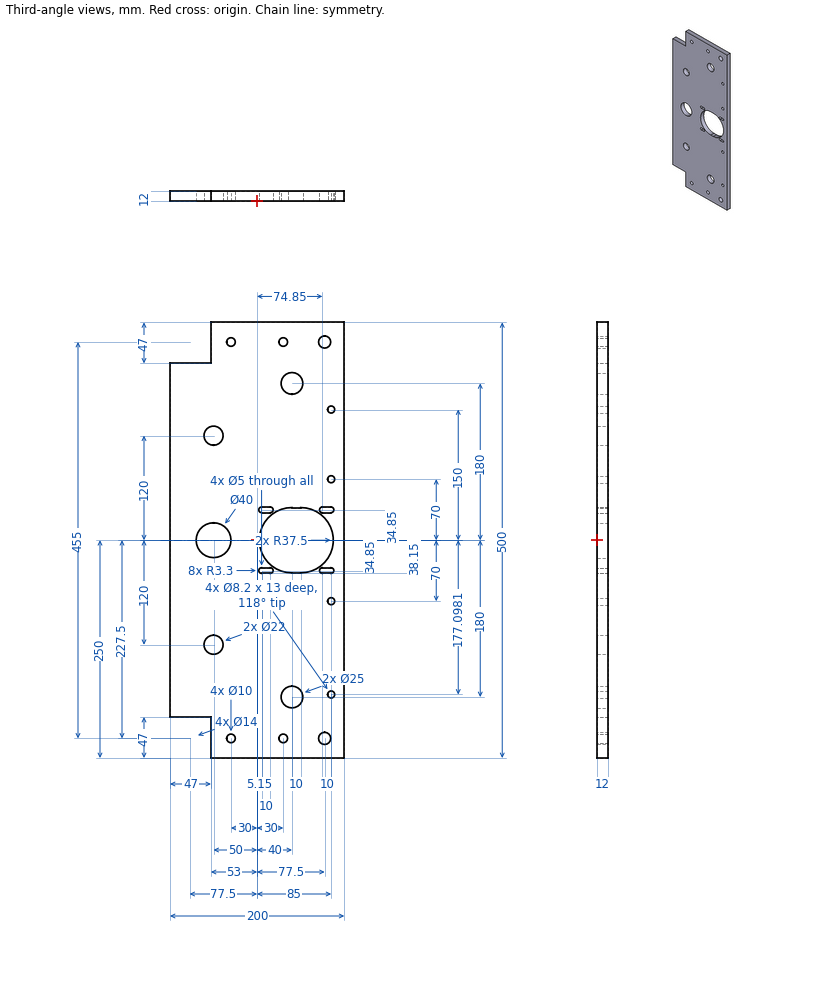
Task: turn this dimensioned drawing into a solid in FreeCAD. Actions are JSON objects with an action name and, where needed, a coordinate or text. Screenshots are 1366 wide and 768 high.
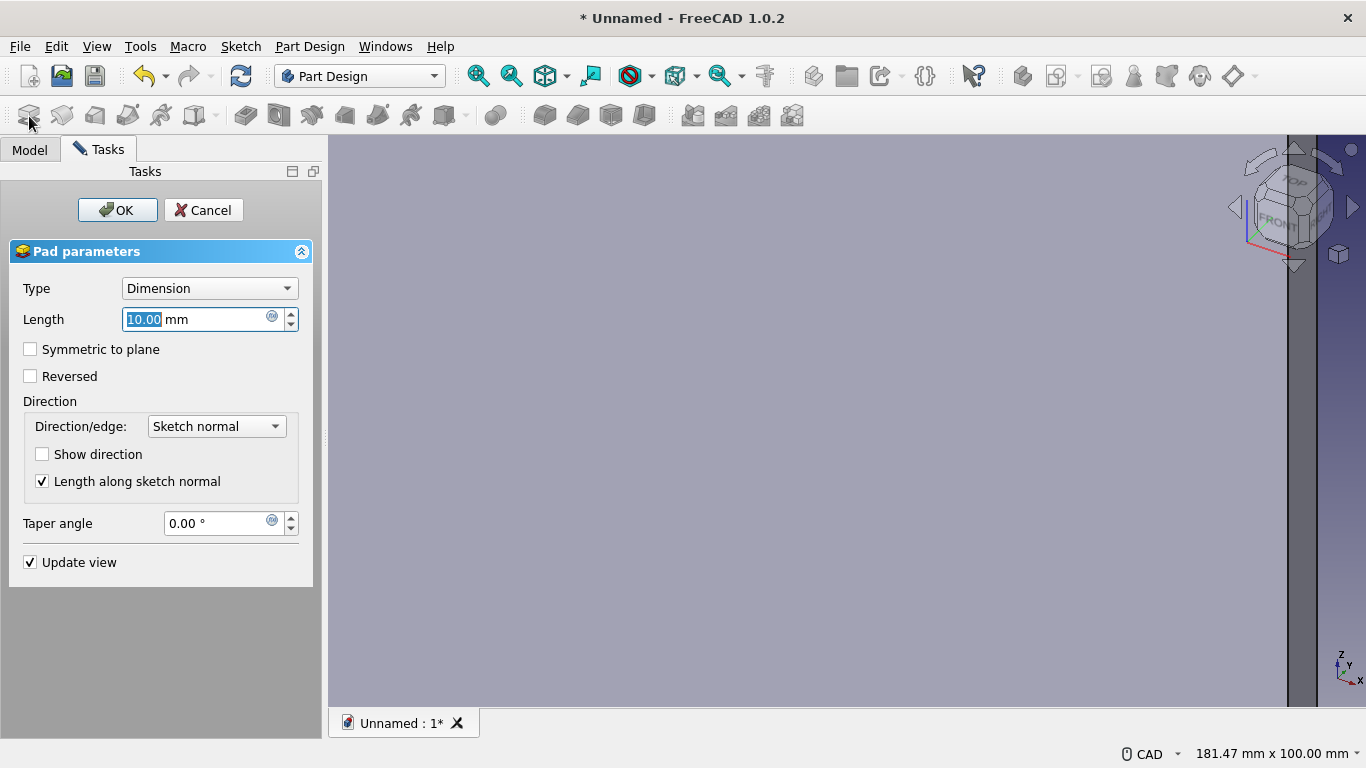
{"action": "type", "text": "12"}
{"action": "key", "text": "Tab"}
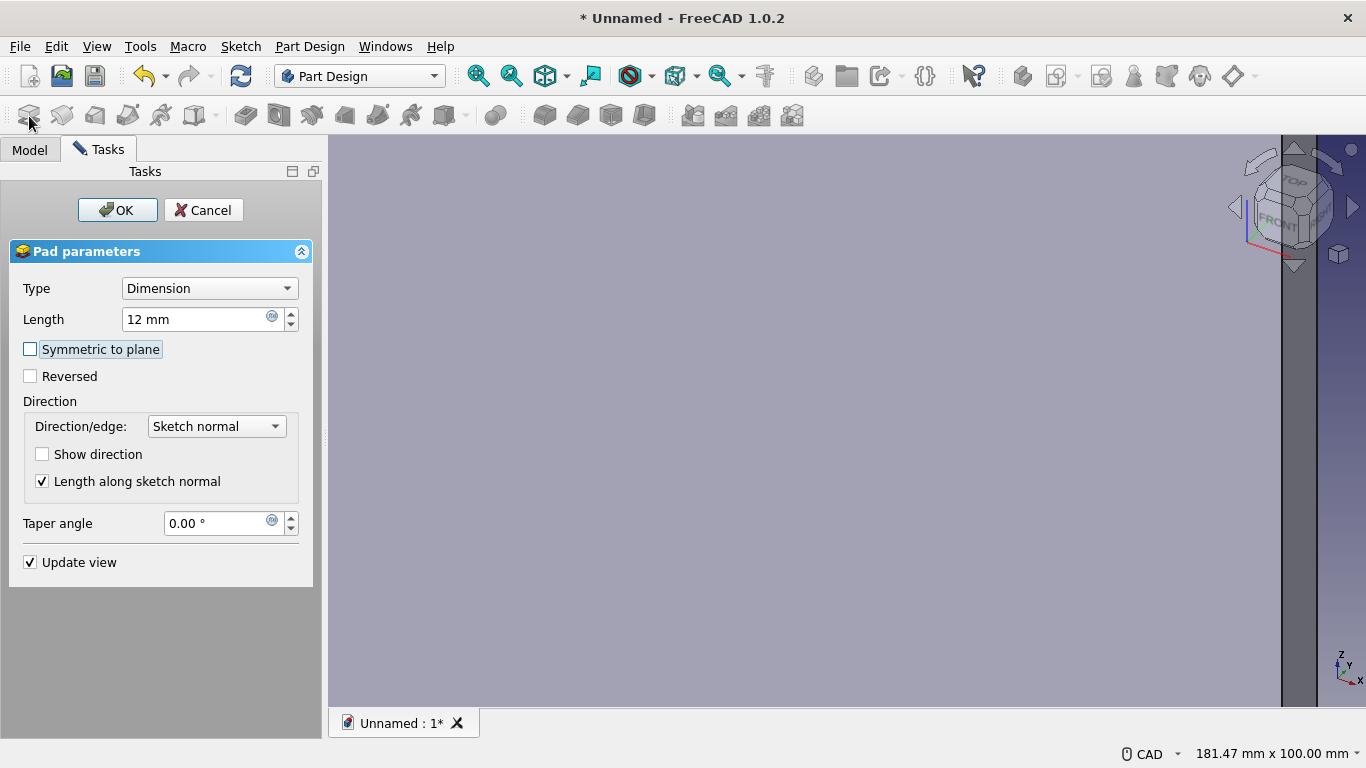
{"action": "left_click", "coordinate": [31, 376]}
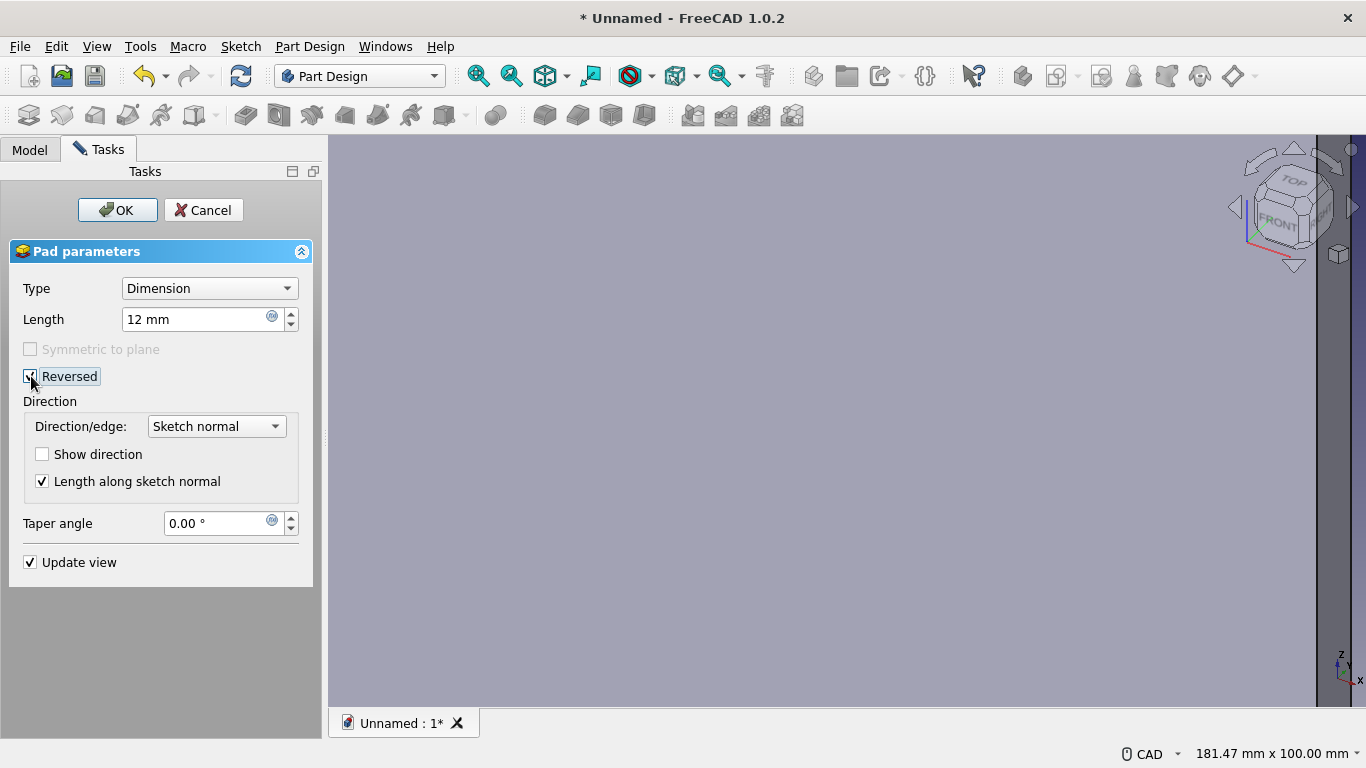
{"action": "left_click", "coordinate": [118, 210]}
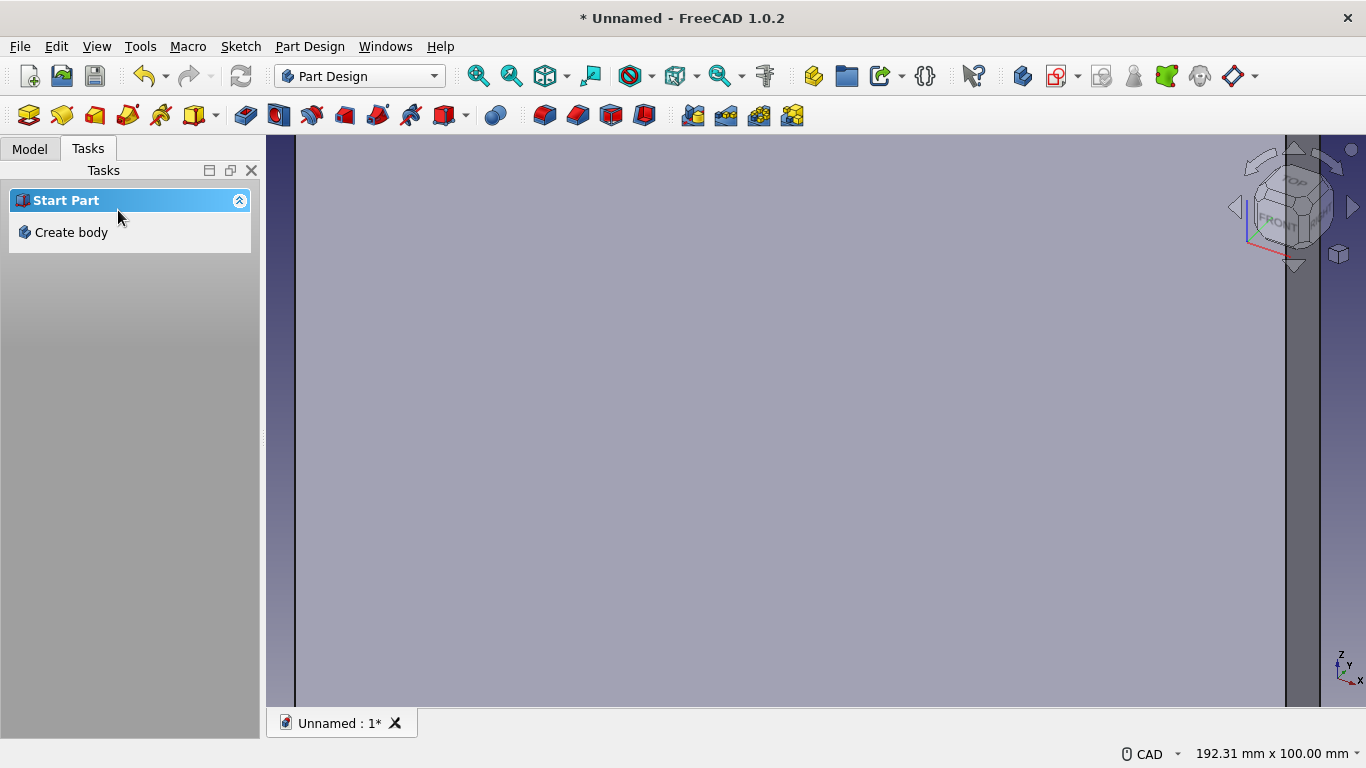
{"action": "key", "text": "v f"}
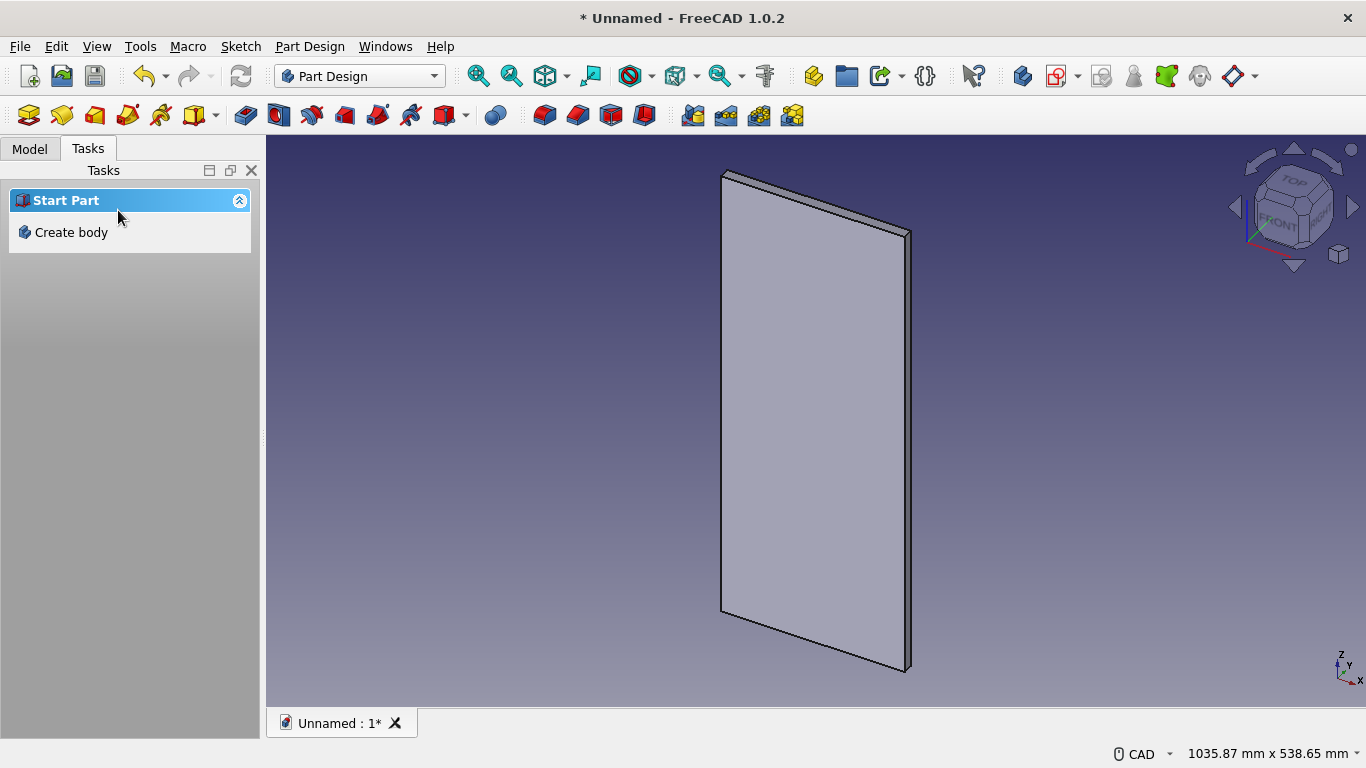
{"action": "key", "text": "4"}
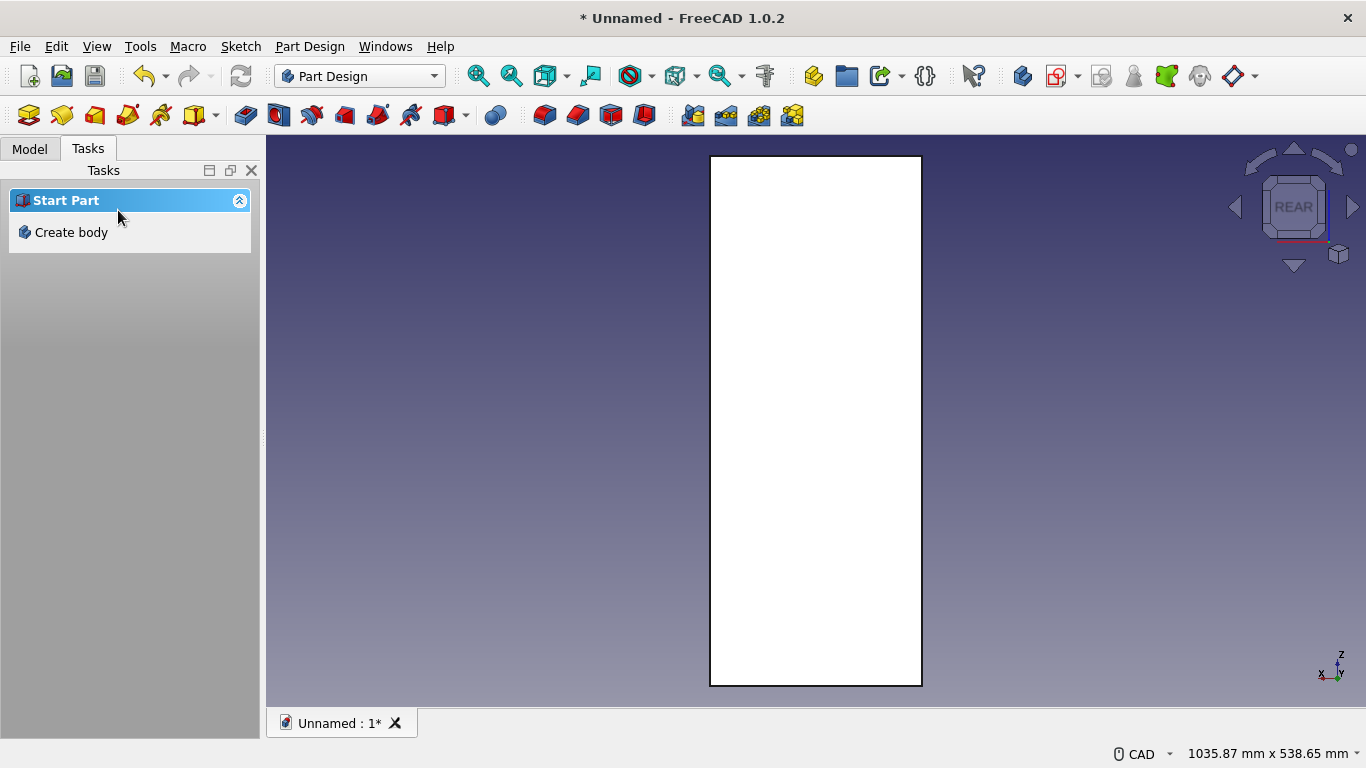
{"action": "left_click", "coordinate": [816, 268]}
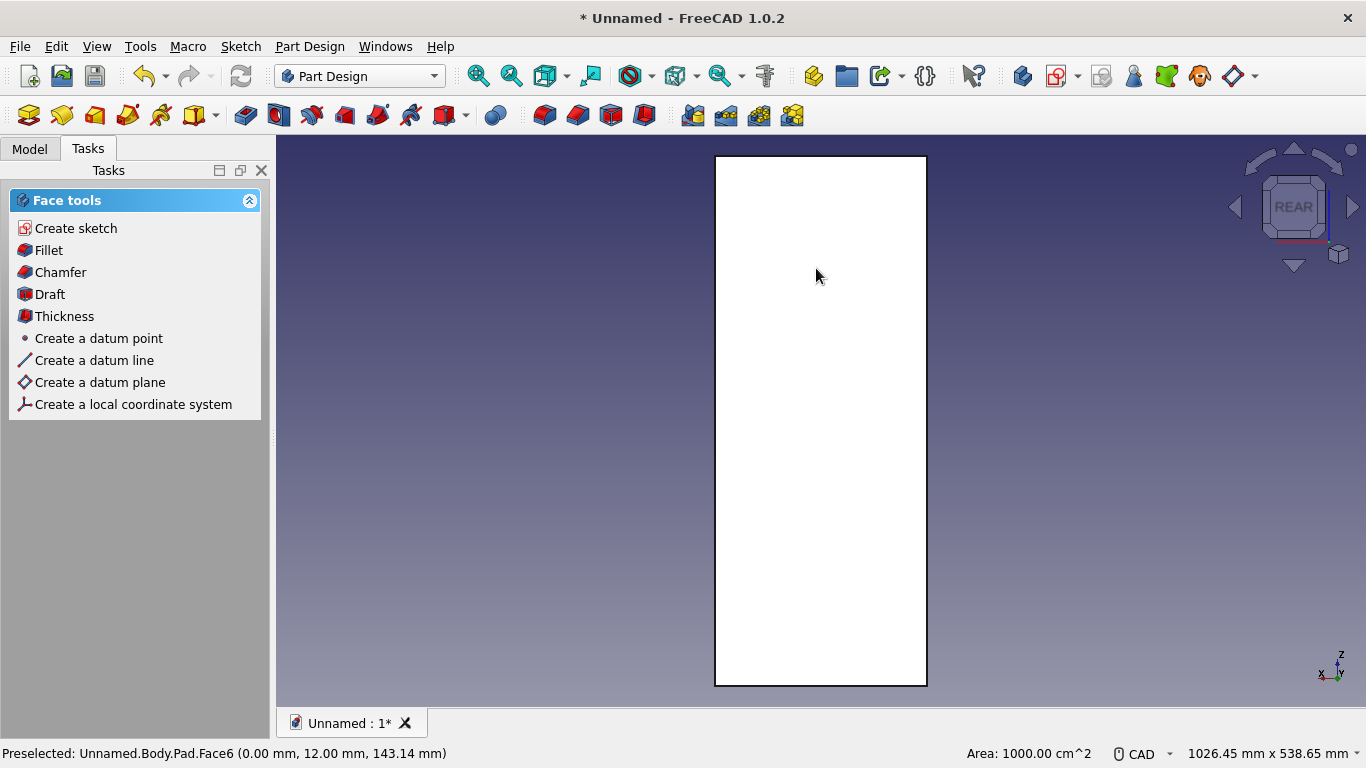
{"action": "left_click", "coordinate": [1056, 76]}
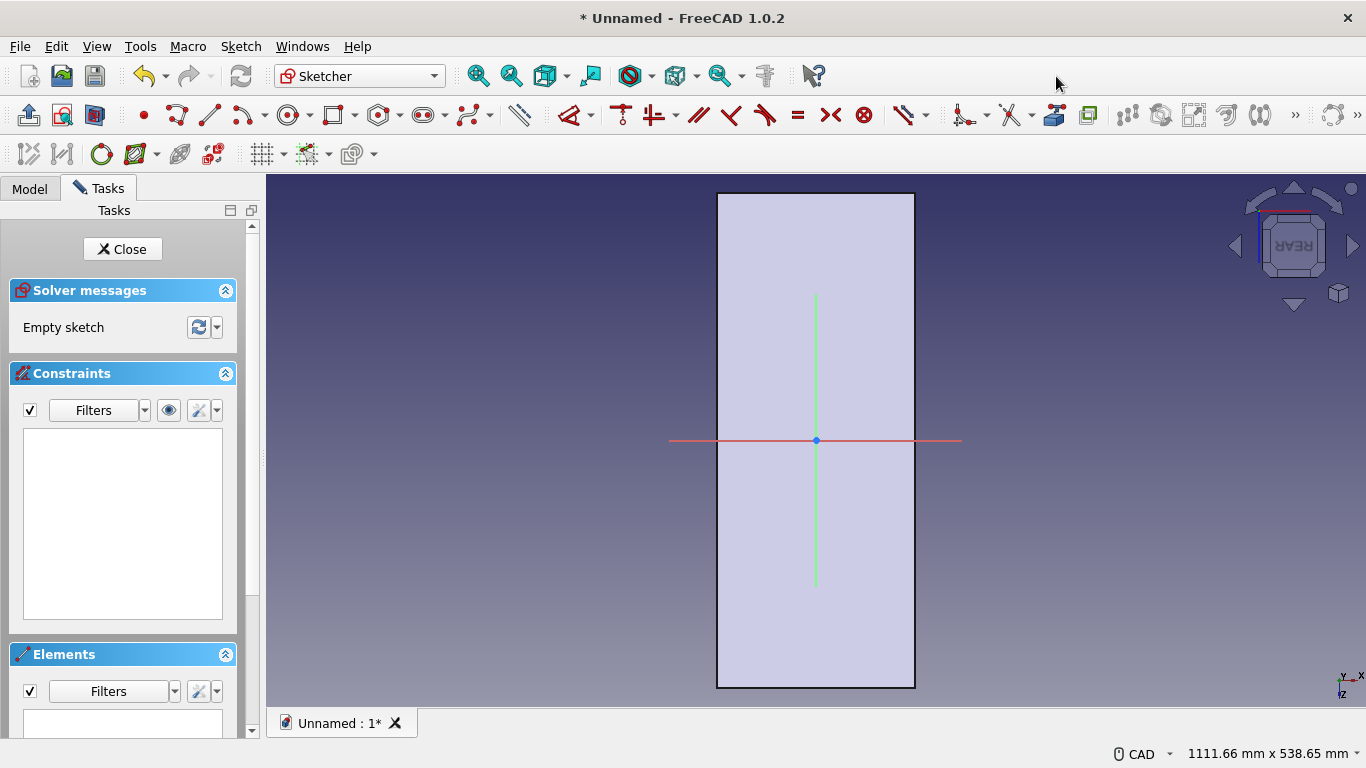
{"action": "key", "text": "g c"}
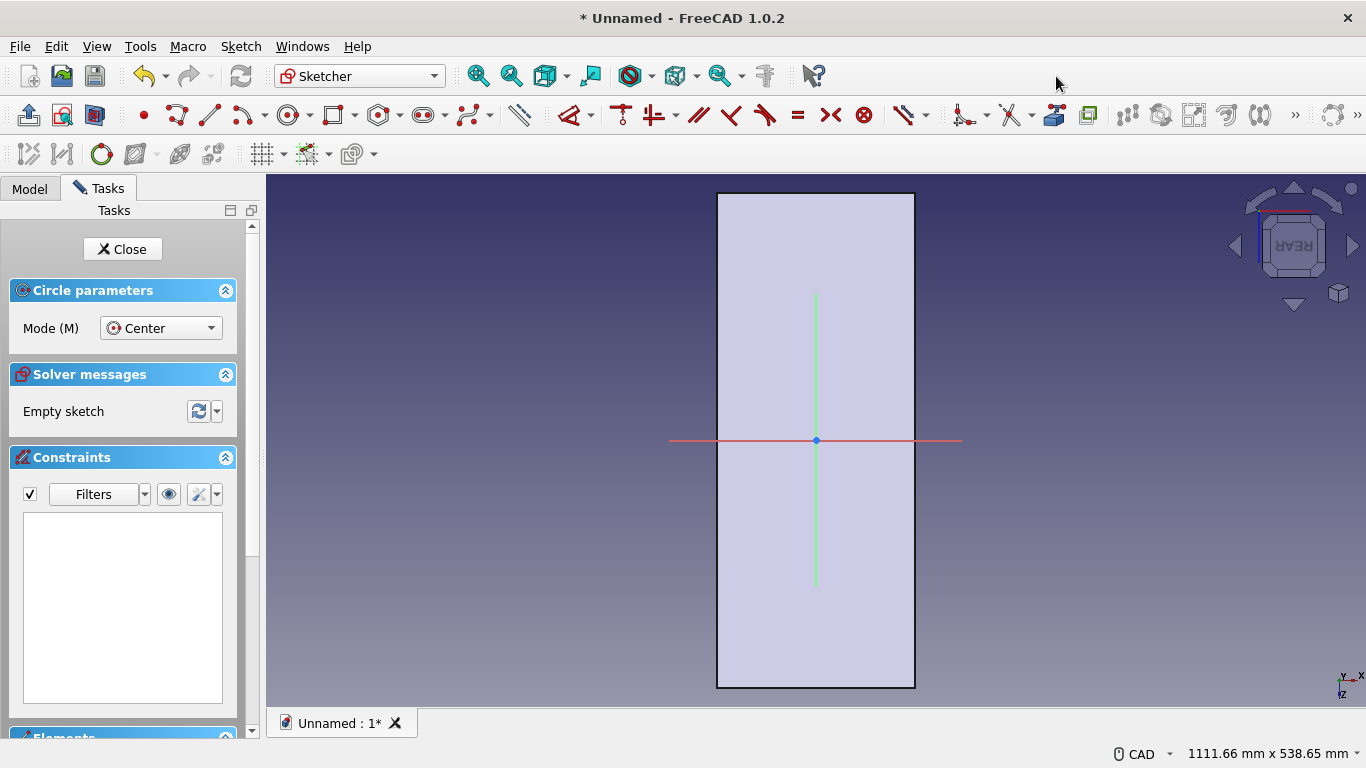
{"action": "left_click", "coordinate": [767, 441]}
{"action": "mouse_move", "coordinate": [773, 422]}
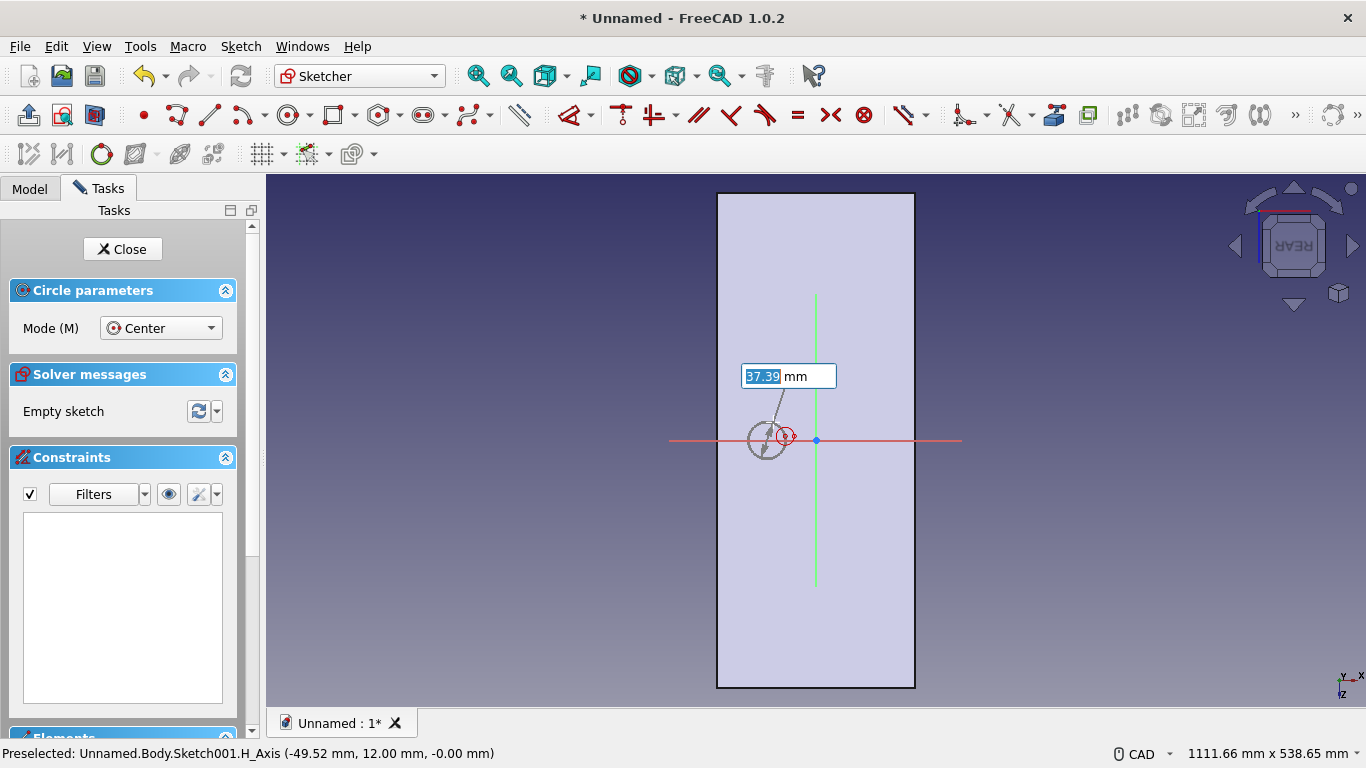
{"action": "type", "text": "40"}
{"action": "key", "text": "Return"}